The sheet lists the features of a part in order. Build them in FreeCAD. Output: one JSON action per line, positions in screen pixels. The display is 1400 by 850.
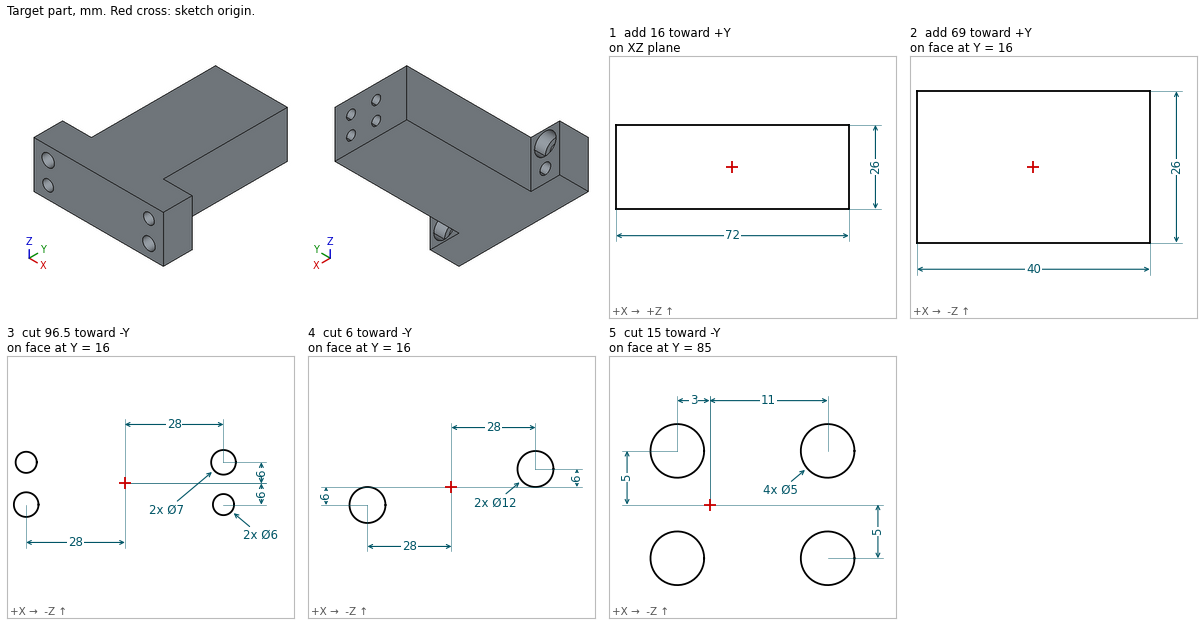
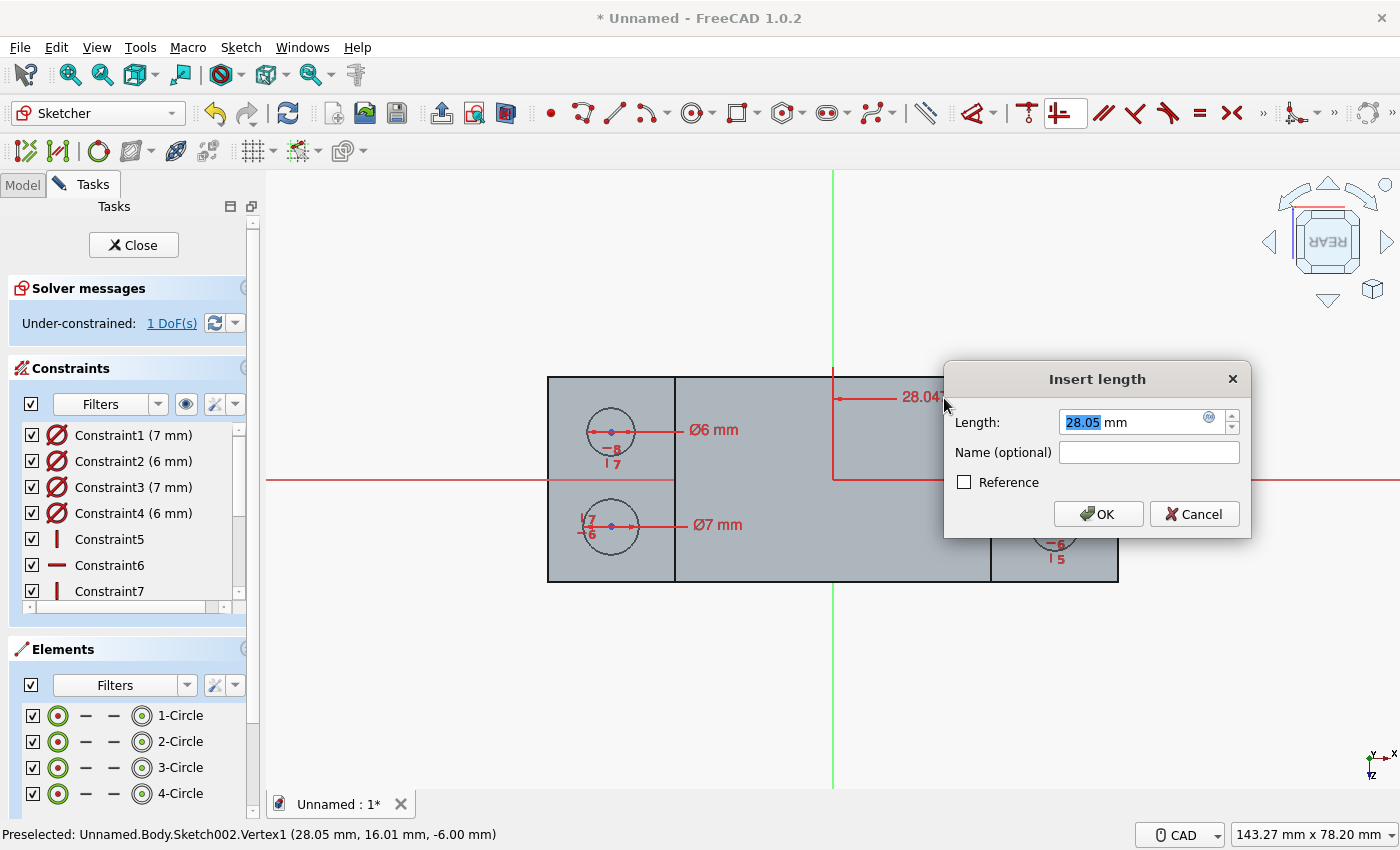
{"action": "type", "text": "28"}
{"action": "key", "text": "Return"}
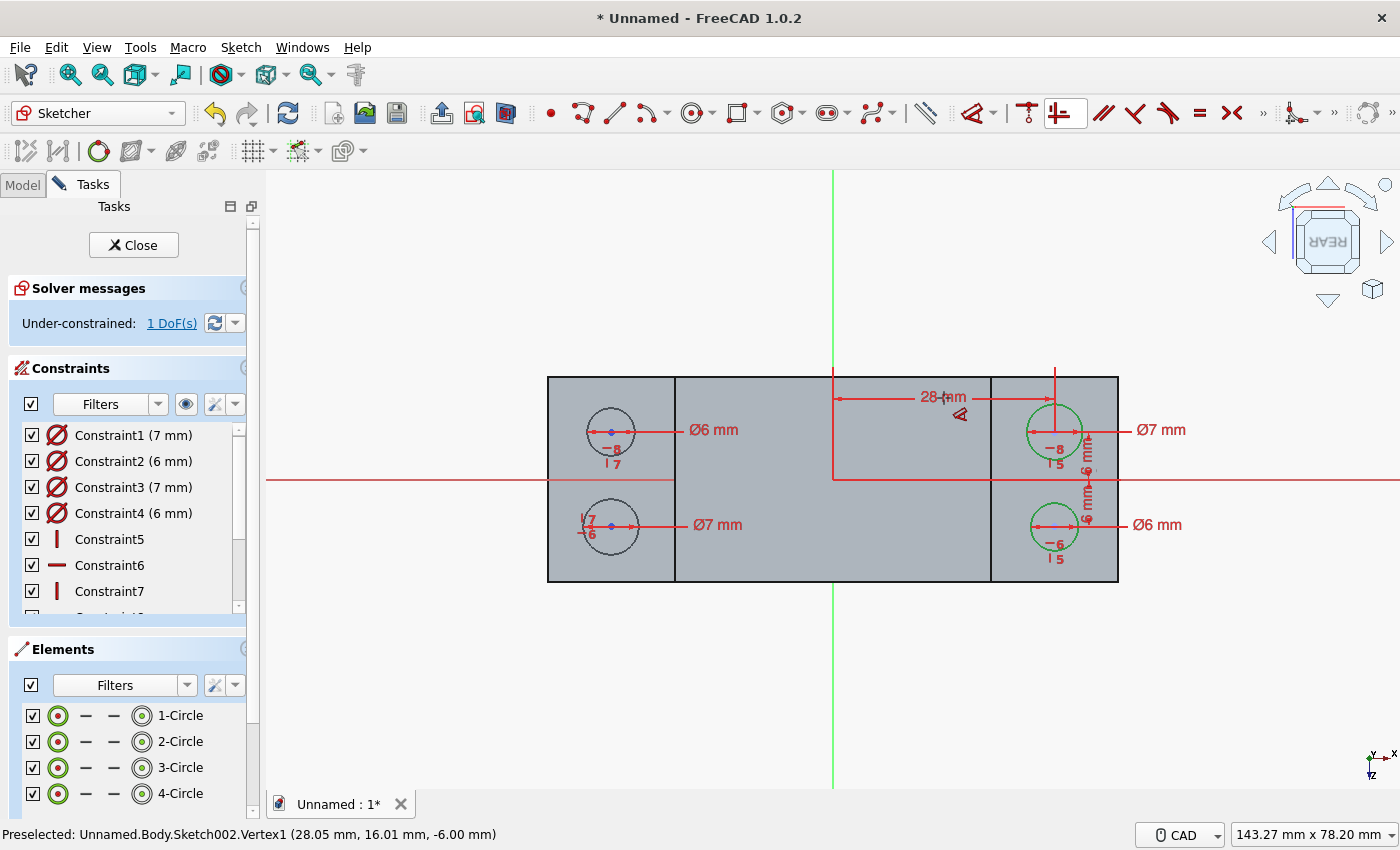
{"action": "left_click", "coordinate": [611, 527]}
{"action": "left_click", "coordinate": [722, 561]}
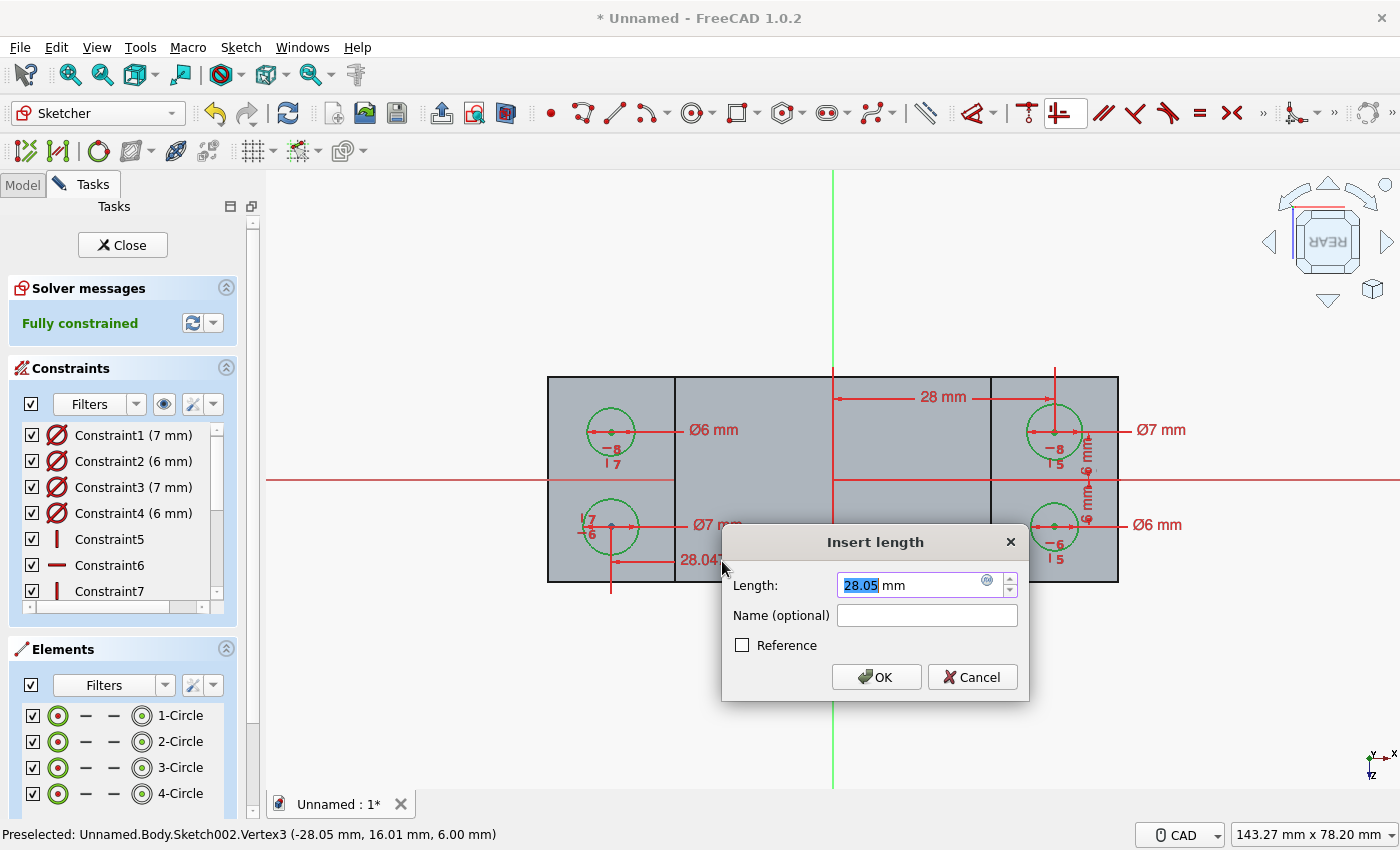
{"action": "type", "text": "28"}
{"action": "key", "text": "Return"}
{"action": "key", "text": "Escape"}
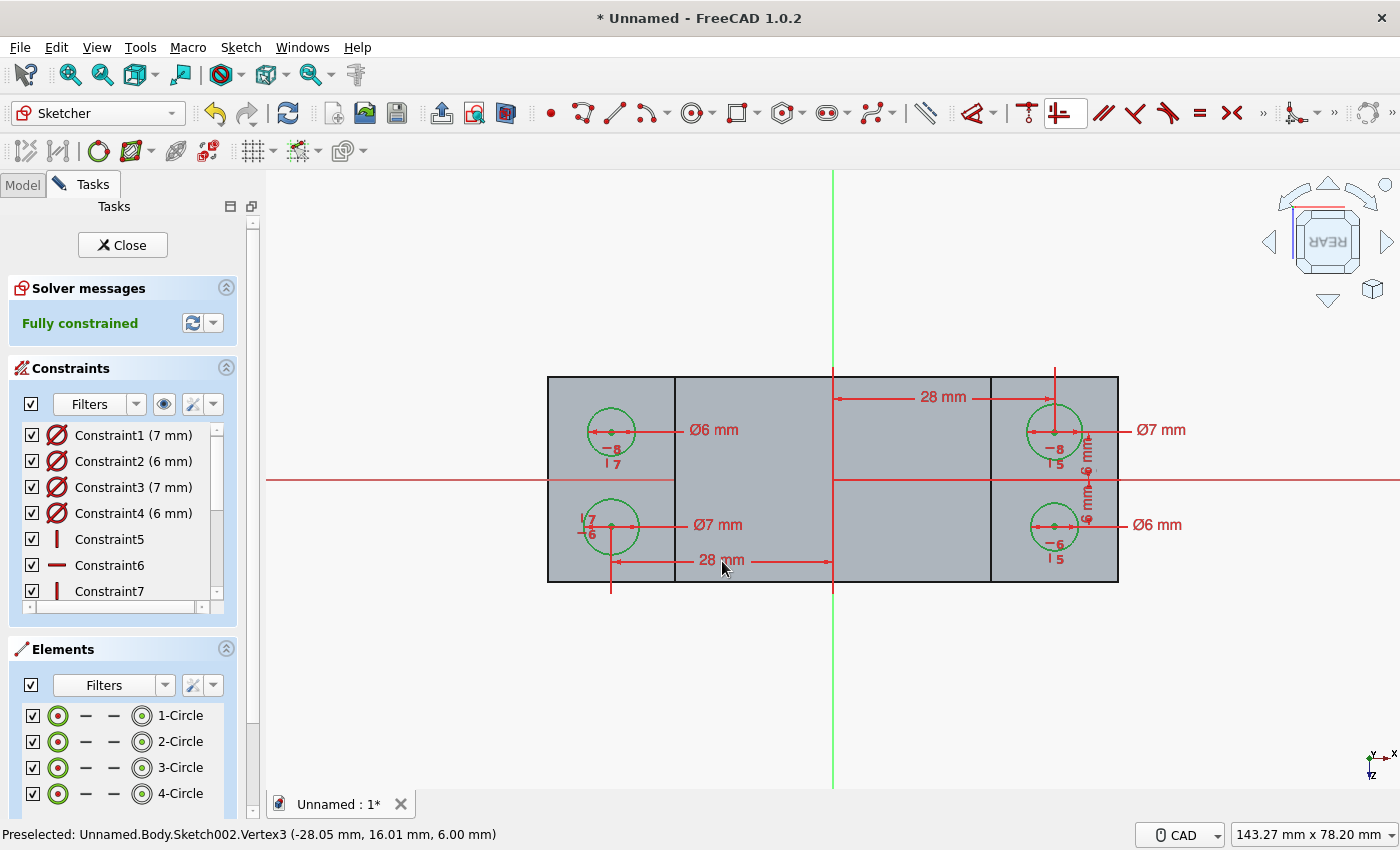
{"action": "left_click", "coordinate": [123, 245]}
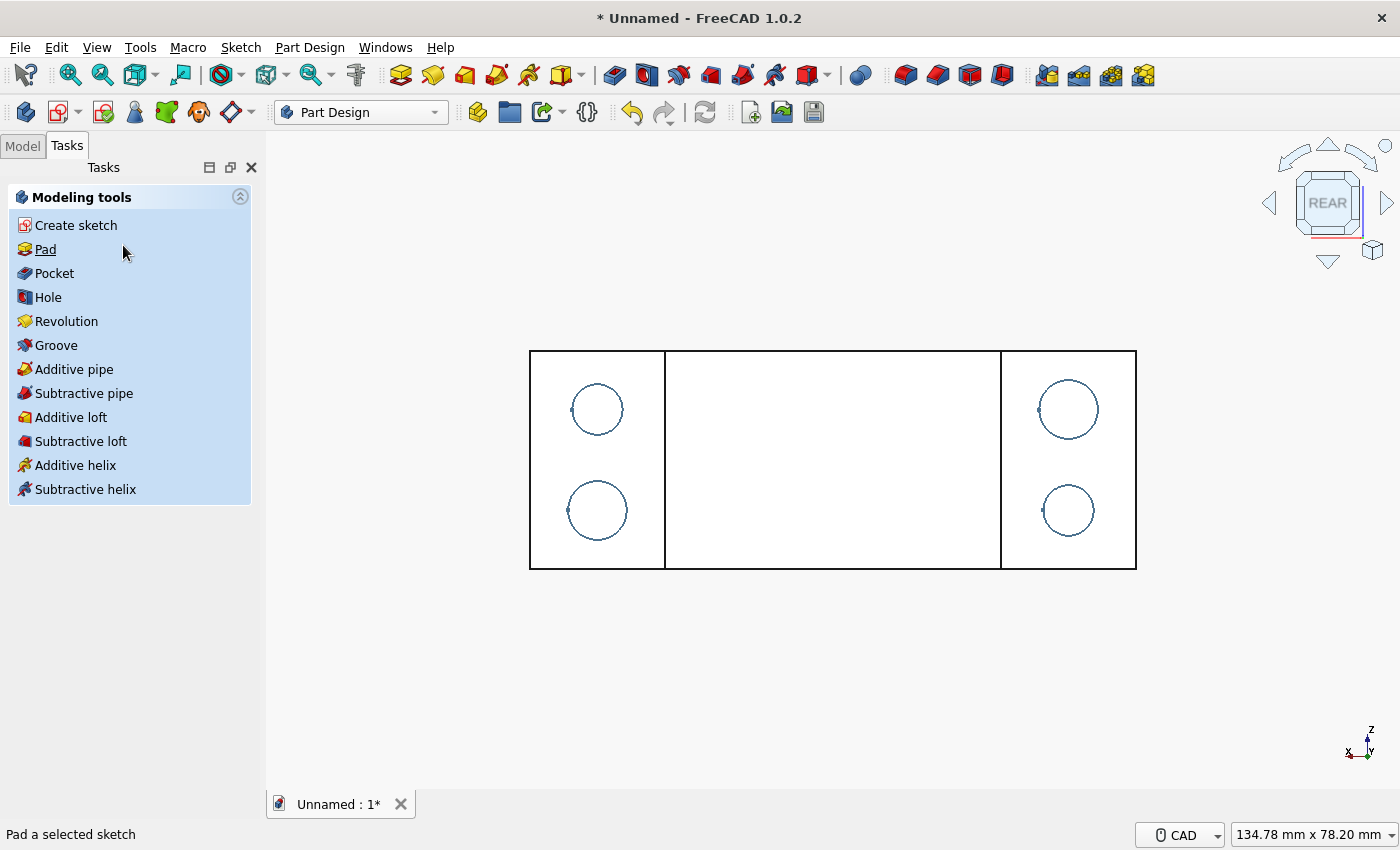
{"action": "left_click", "coordinate": [616, 76]}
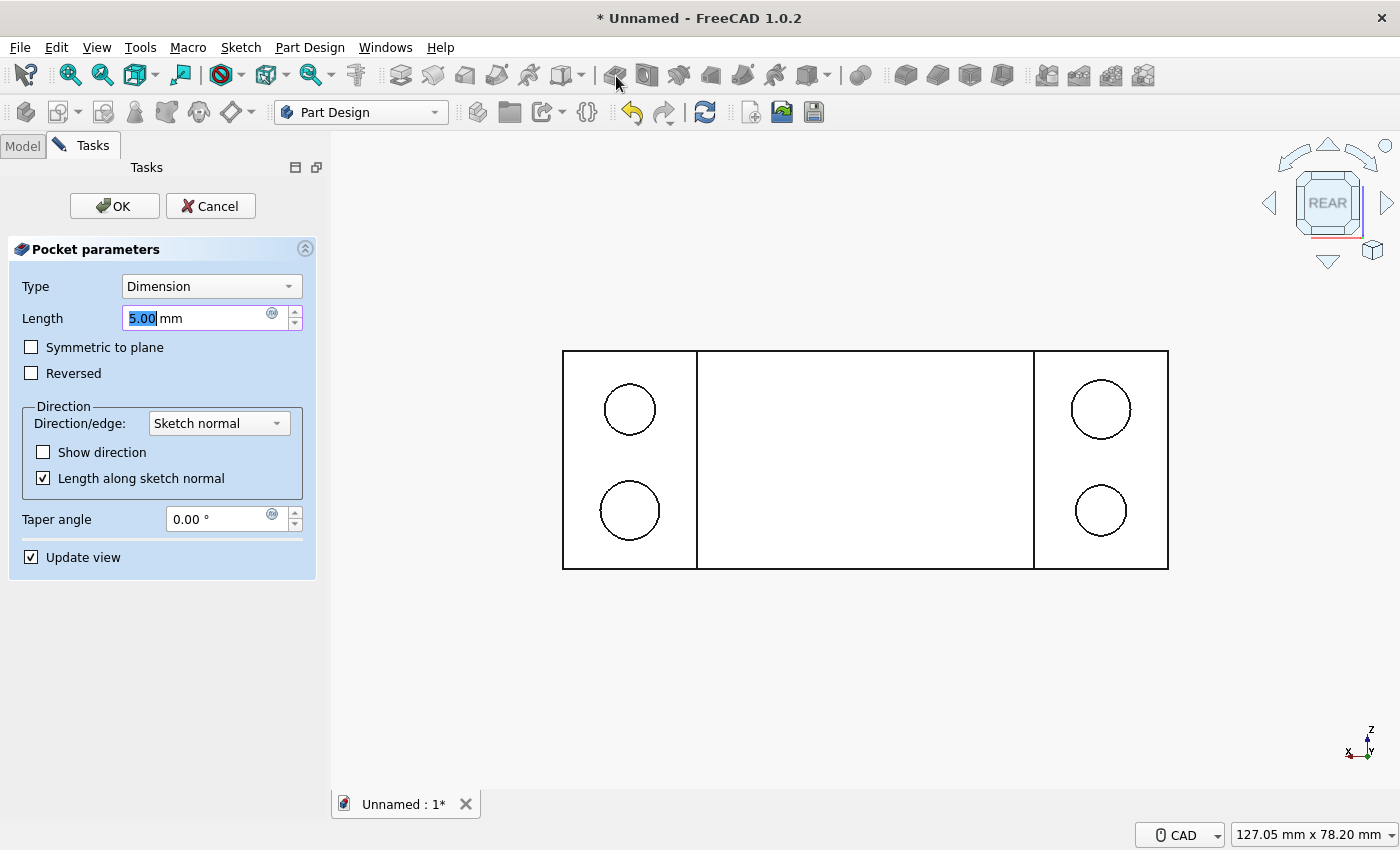
{"action": "type", "text": "96.5"}
{"action": "key", "text": "Tab"}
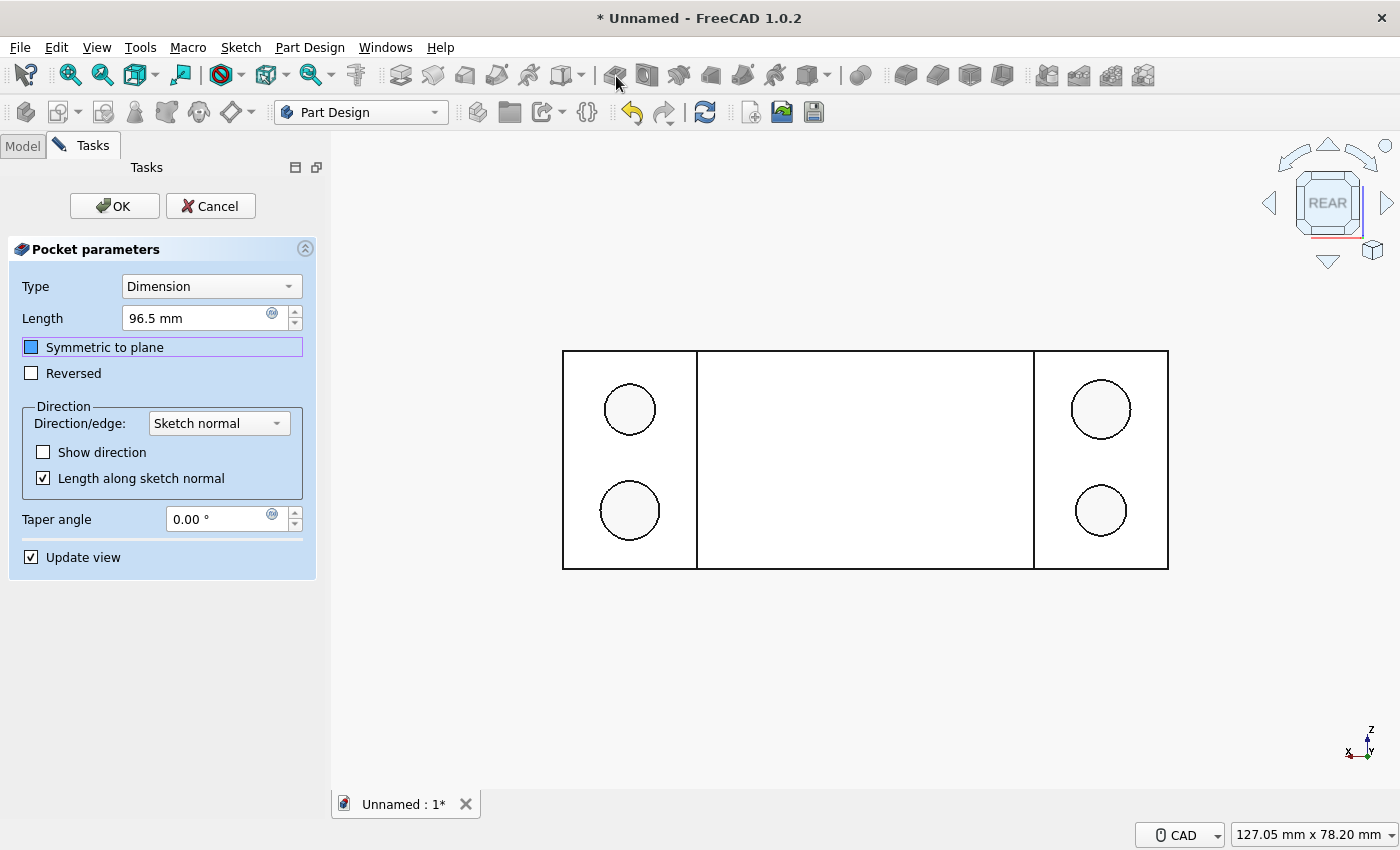
{"action": "left_click", "coordinate": [115, 206]}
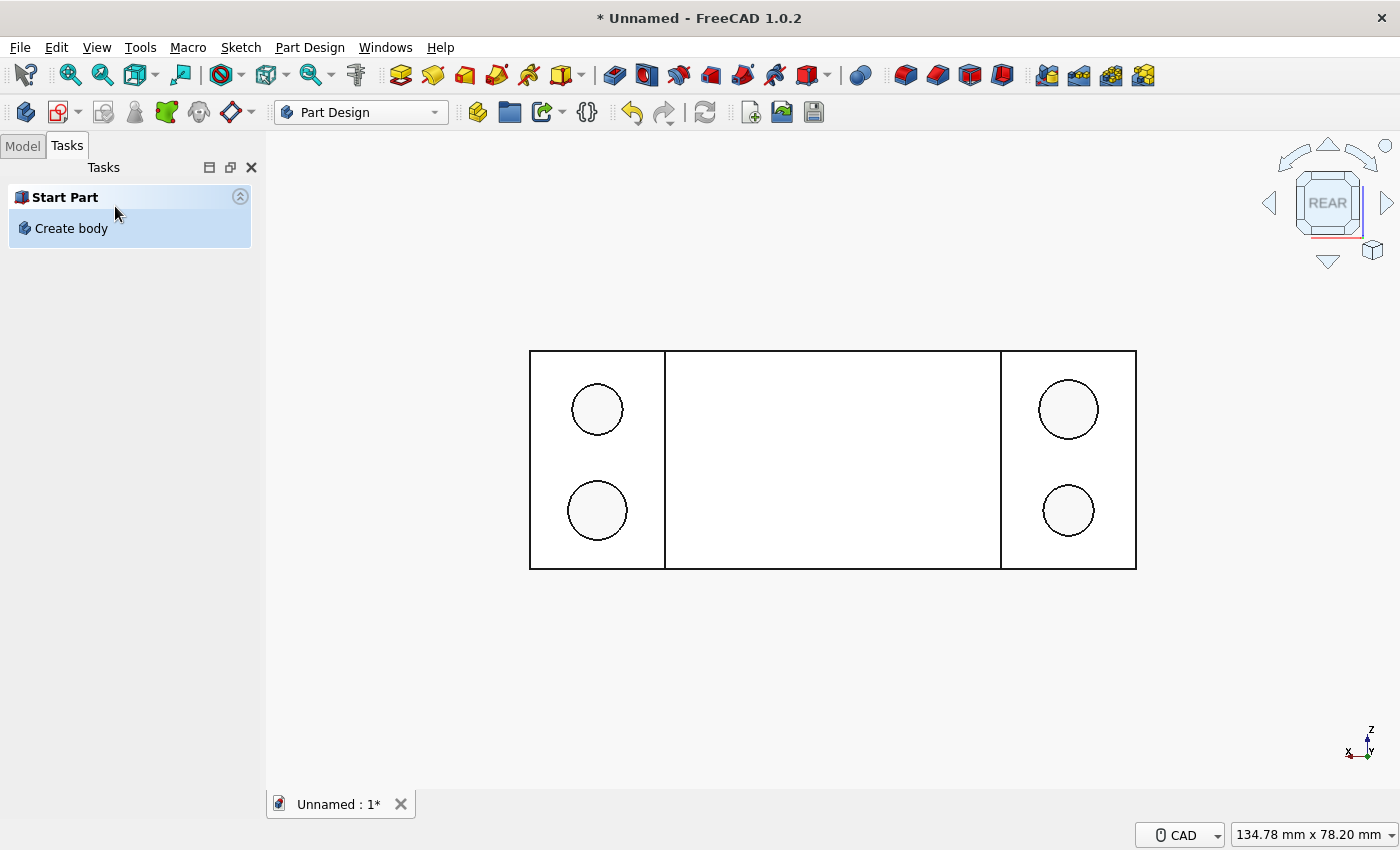
{"action": "left_click", "coordinate": [559, 459]}